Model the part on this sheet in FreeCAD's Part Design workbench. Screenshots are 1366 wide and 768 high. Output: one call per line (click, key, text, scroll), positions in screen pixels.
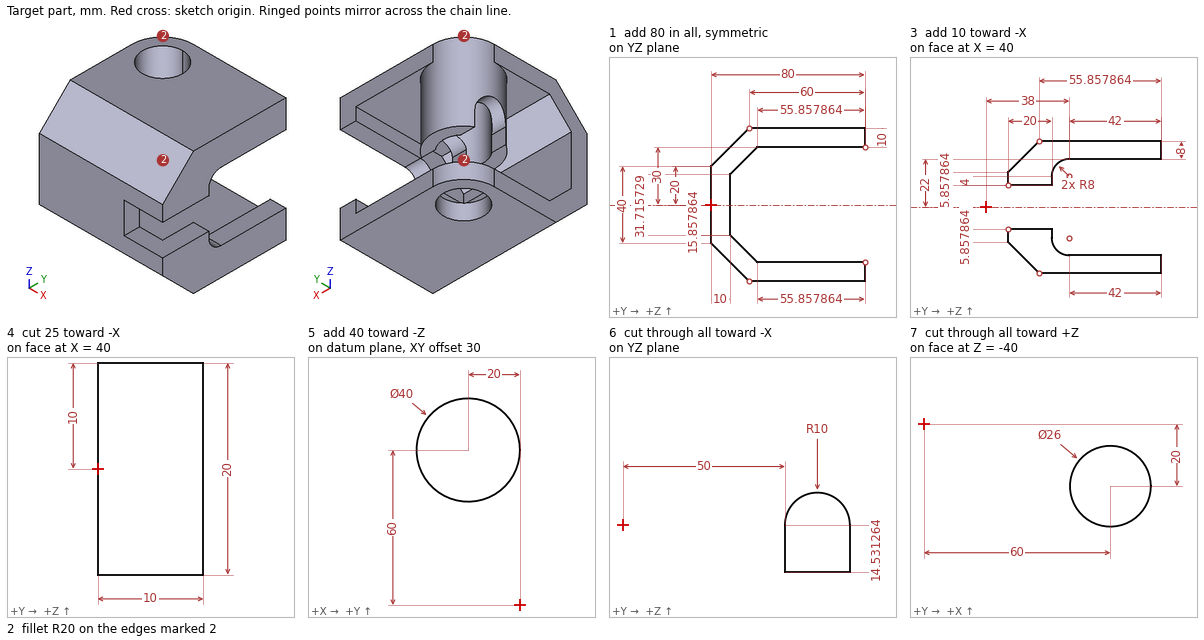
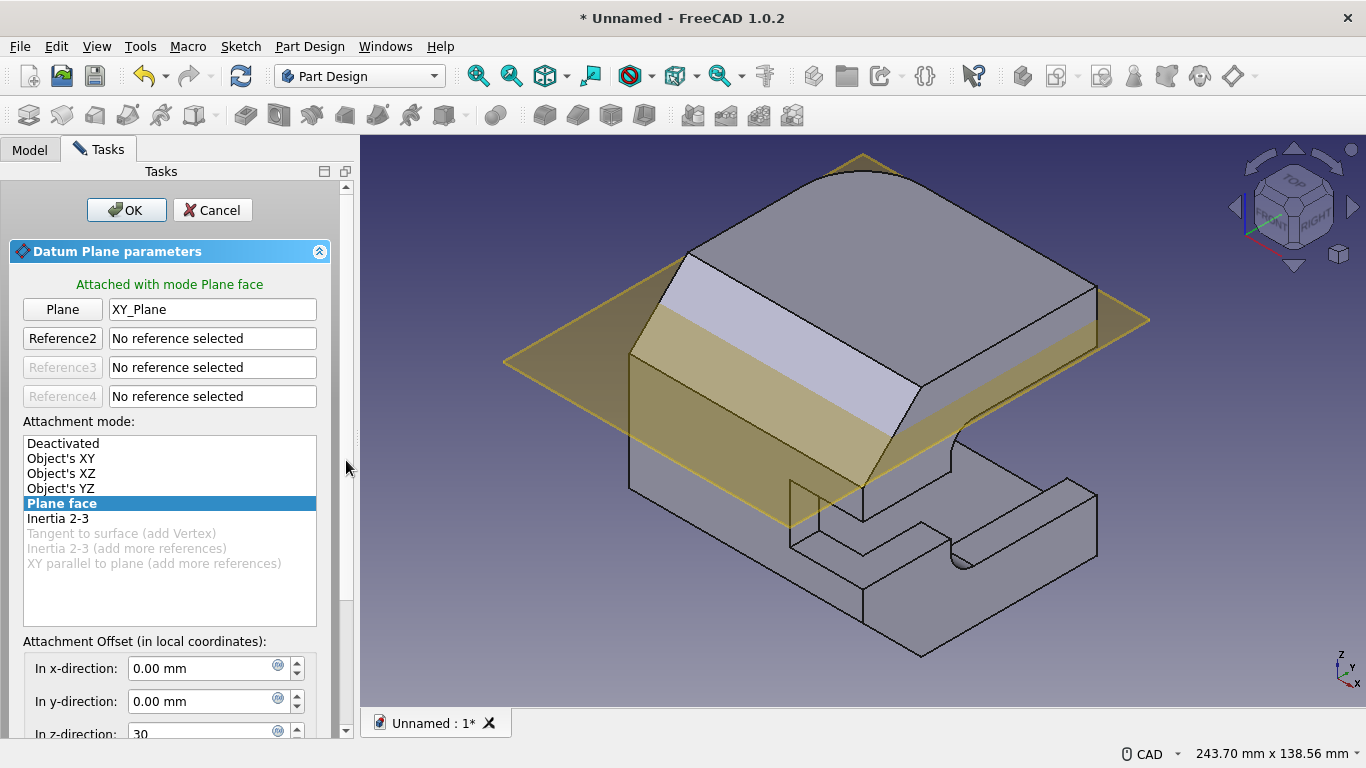
click(127, 210)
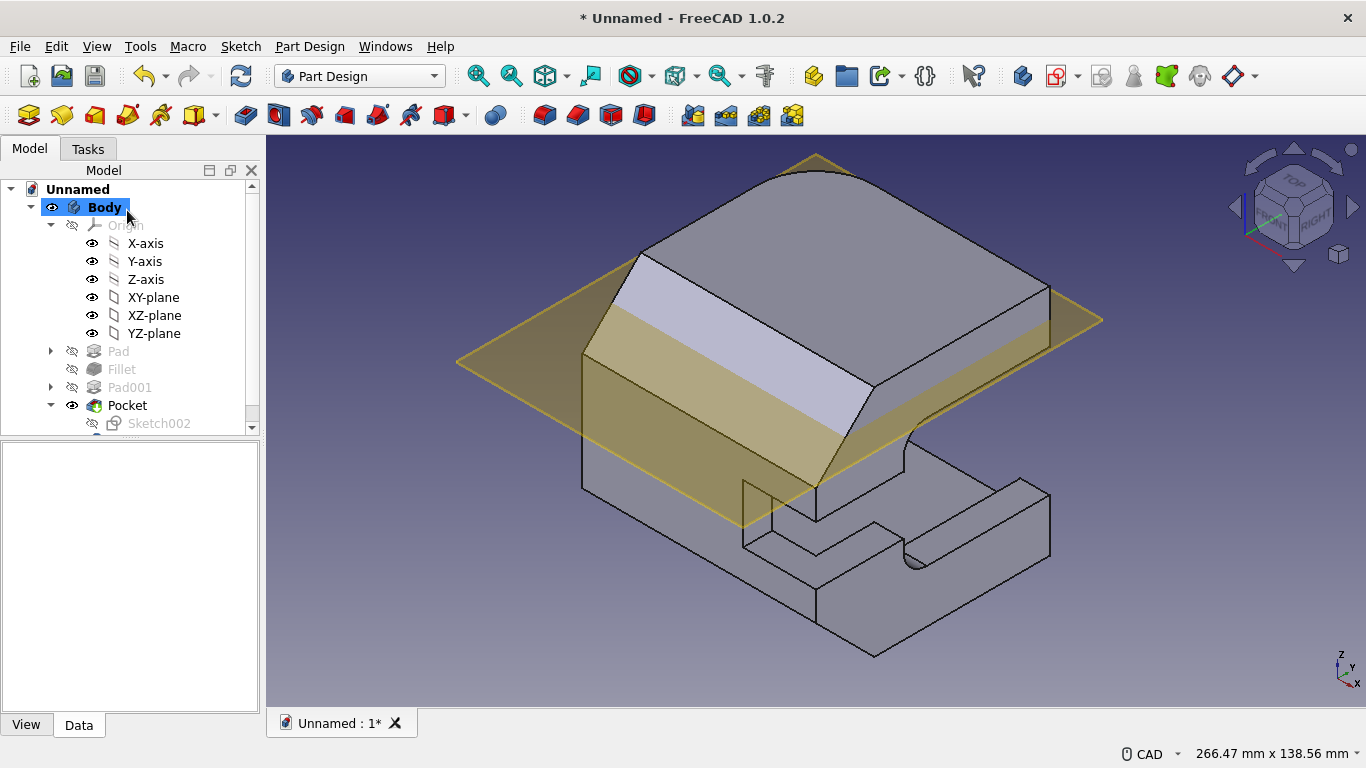
scroll(101, 311, down, 3)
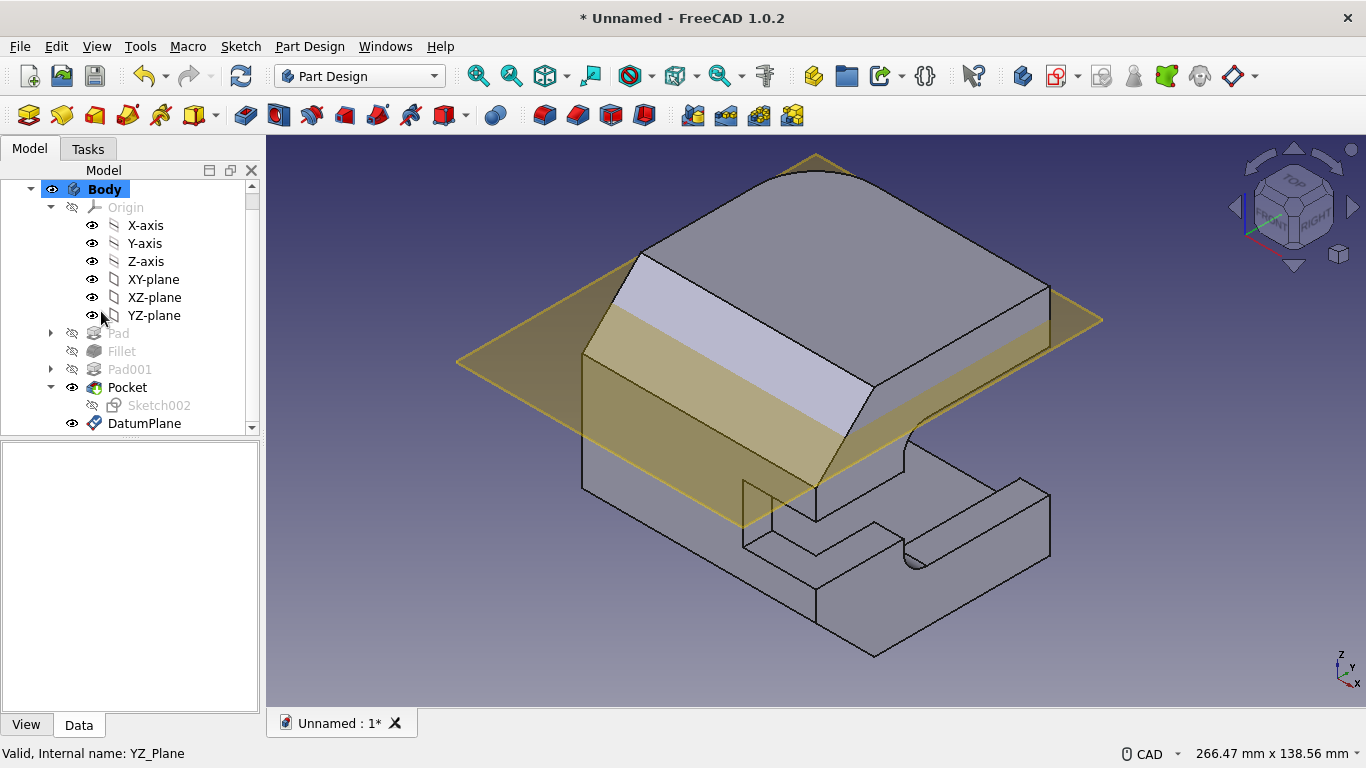
click(117, 423)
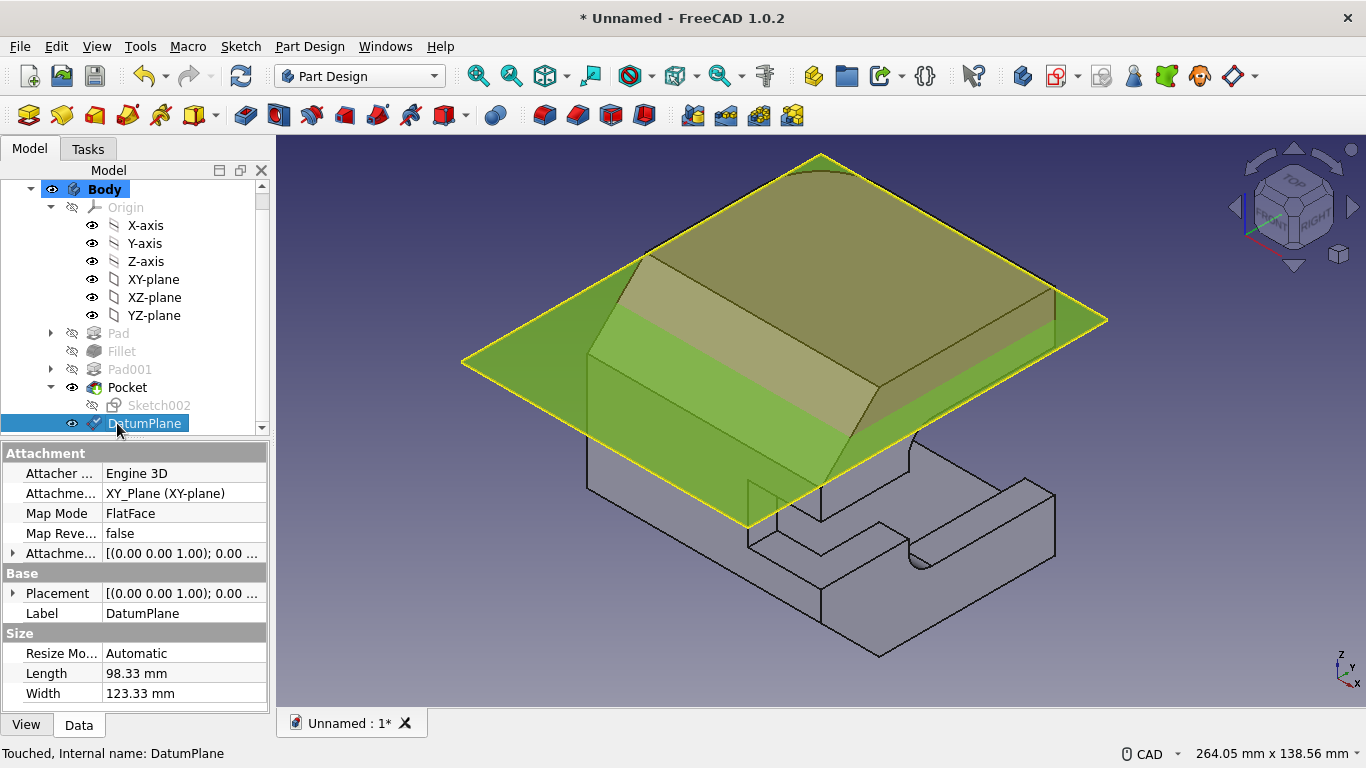
click(1056, 76)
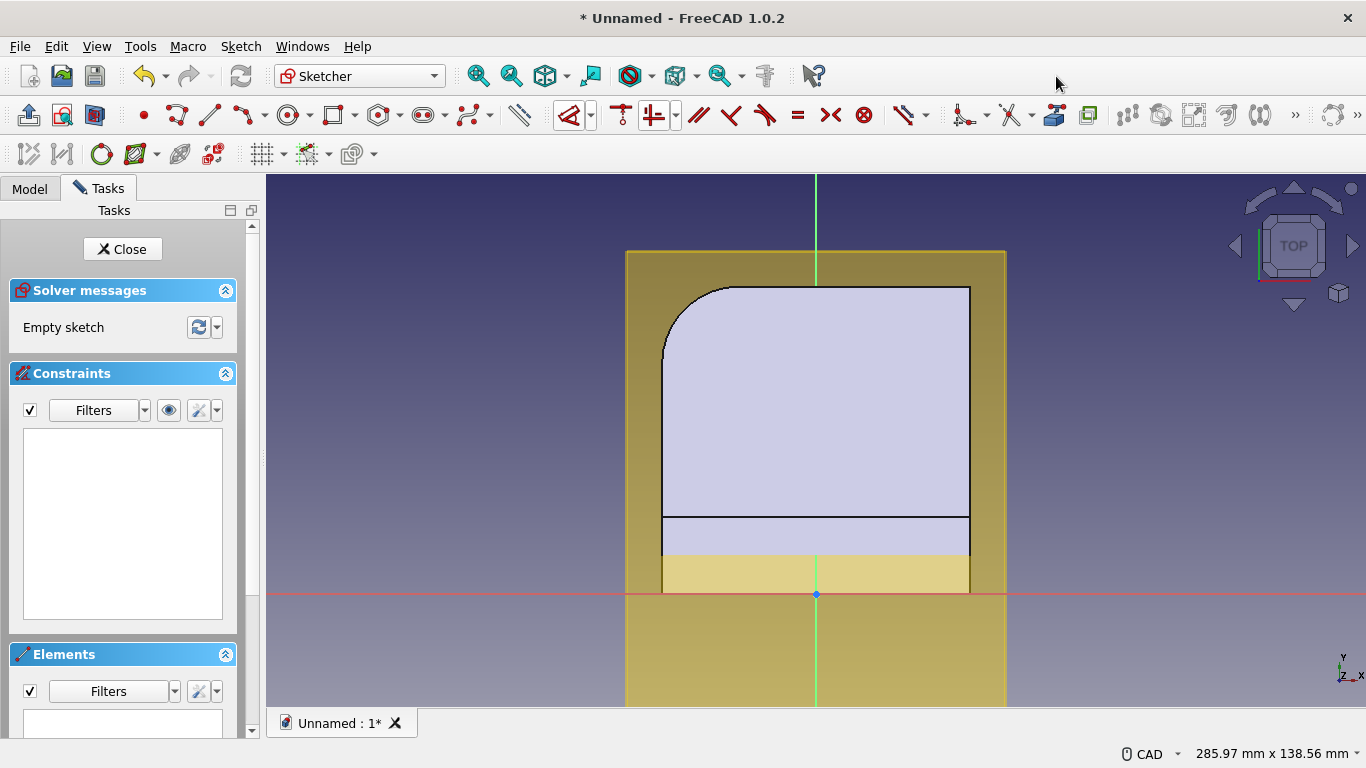
key(q)
key(s)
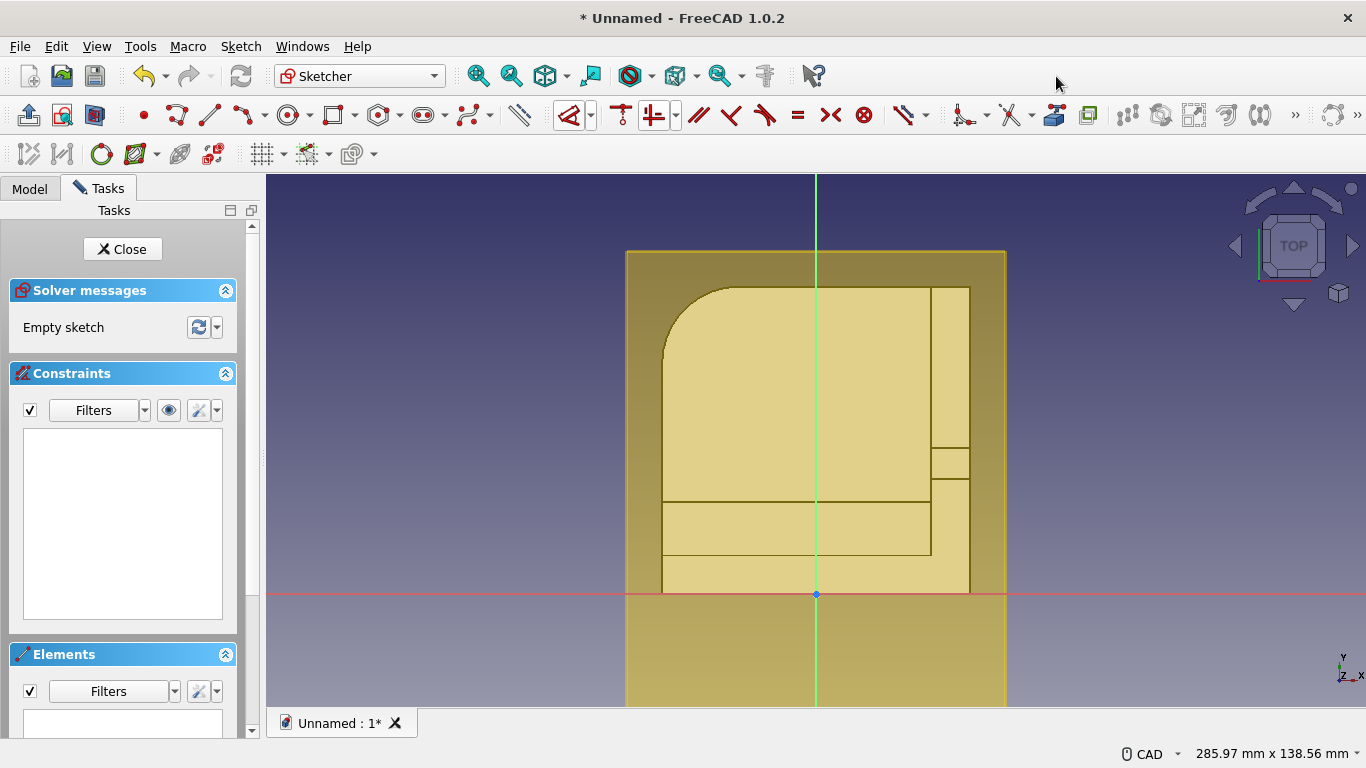
click(288, 116)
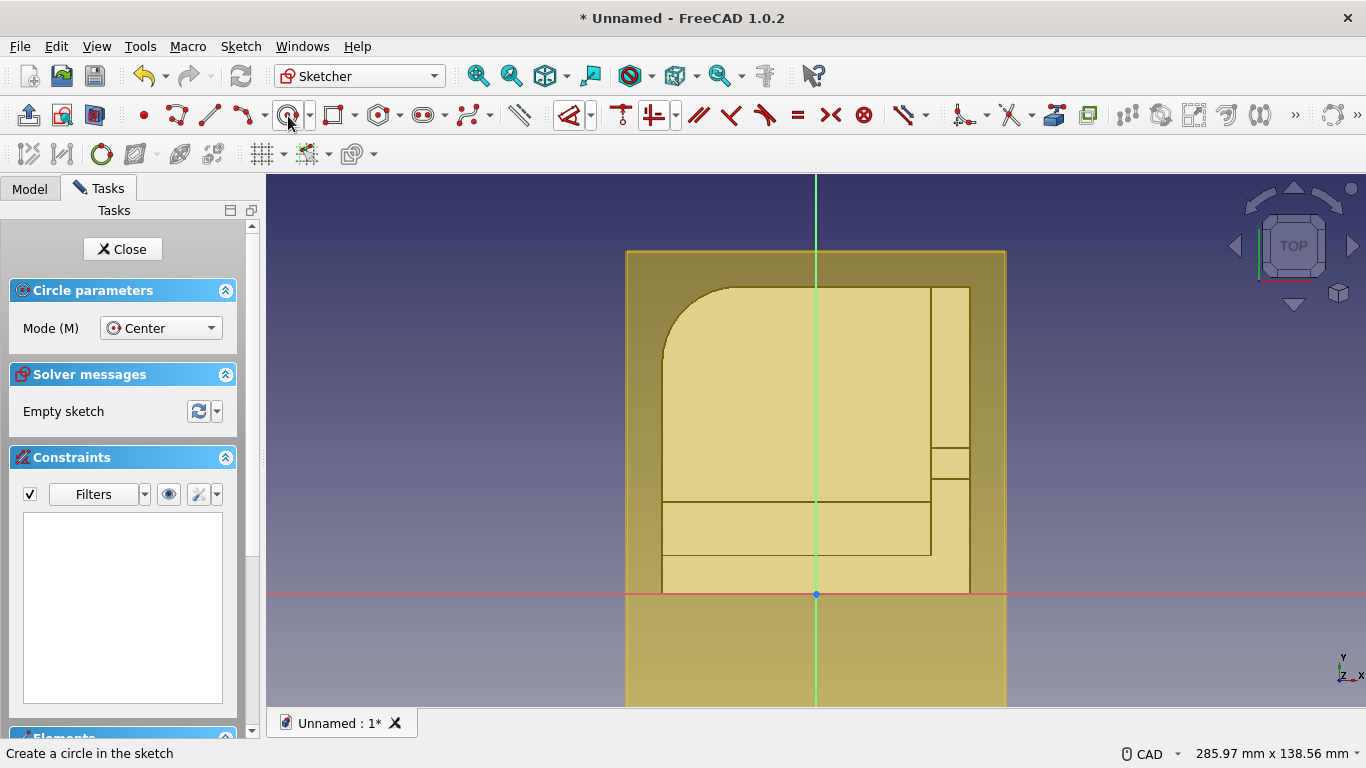
click(739, 364)
move(793, 309)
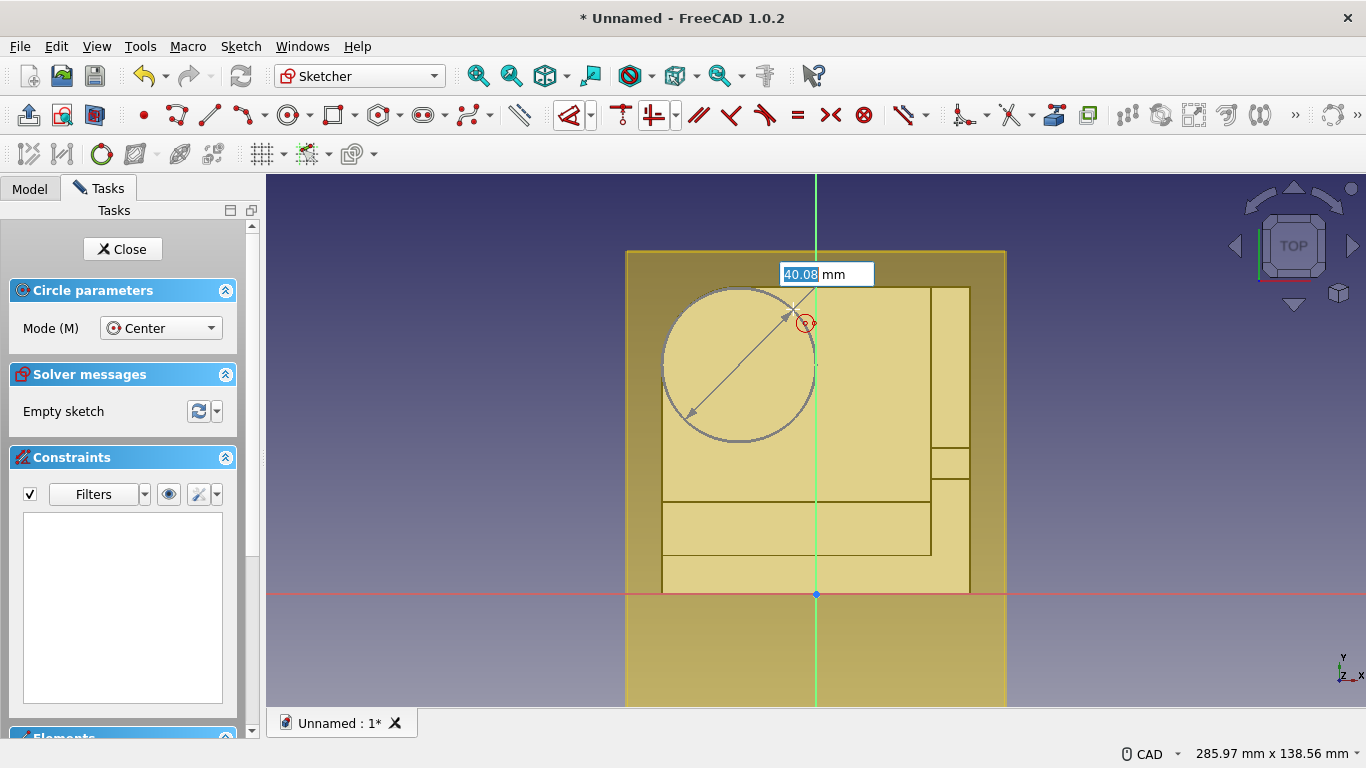
text(40)
key(Return)
key(Escape)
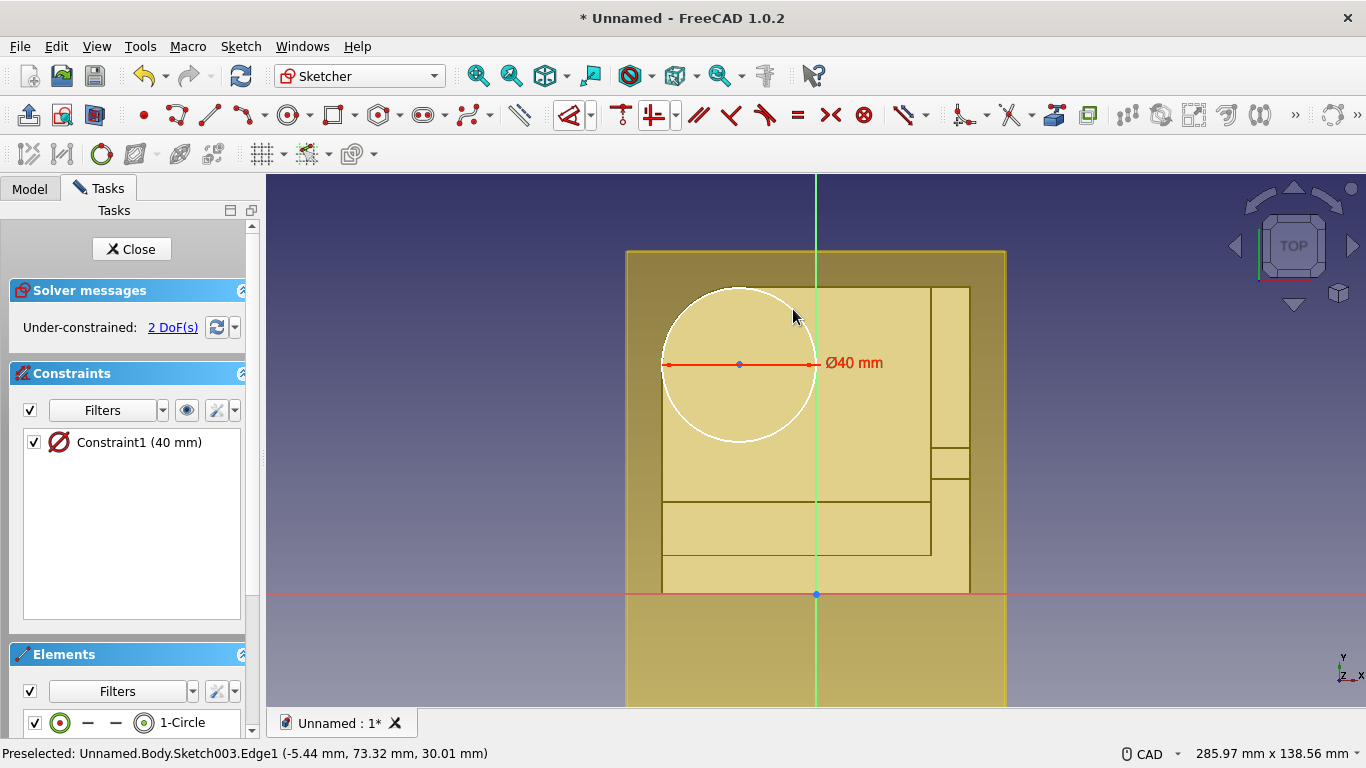
click(739, 365)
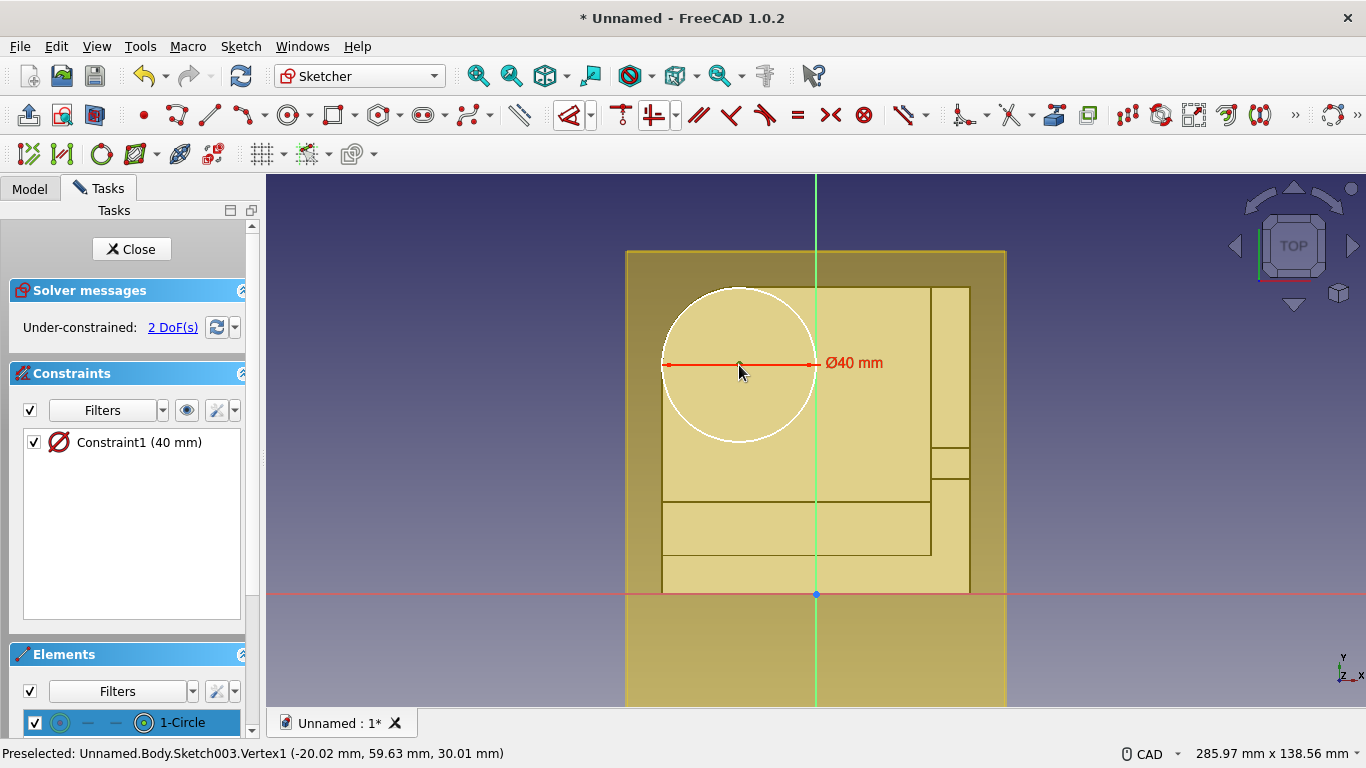
key(l)